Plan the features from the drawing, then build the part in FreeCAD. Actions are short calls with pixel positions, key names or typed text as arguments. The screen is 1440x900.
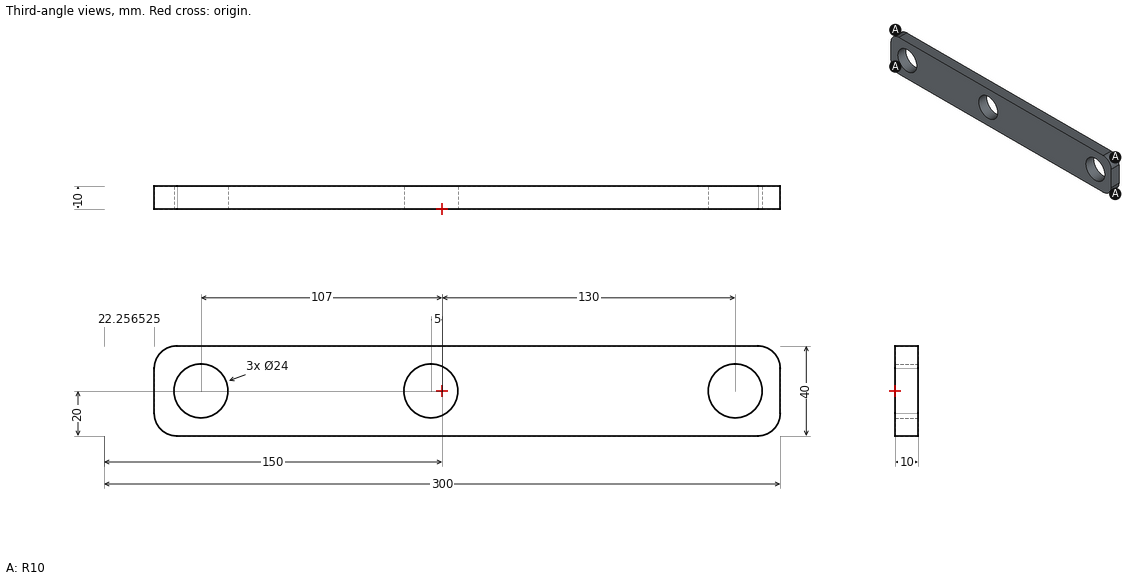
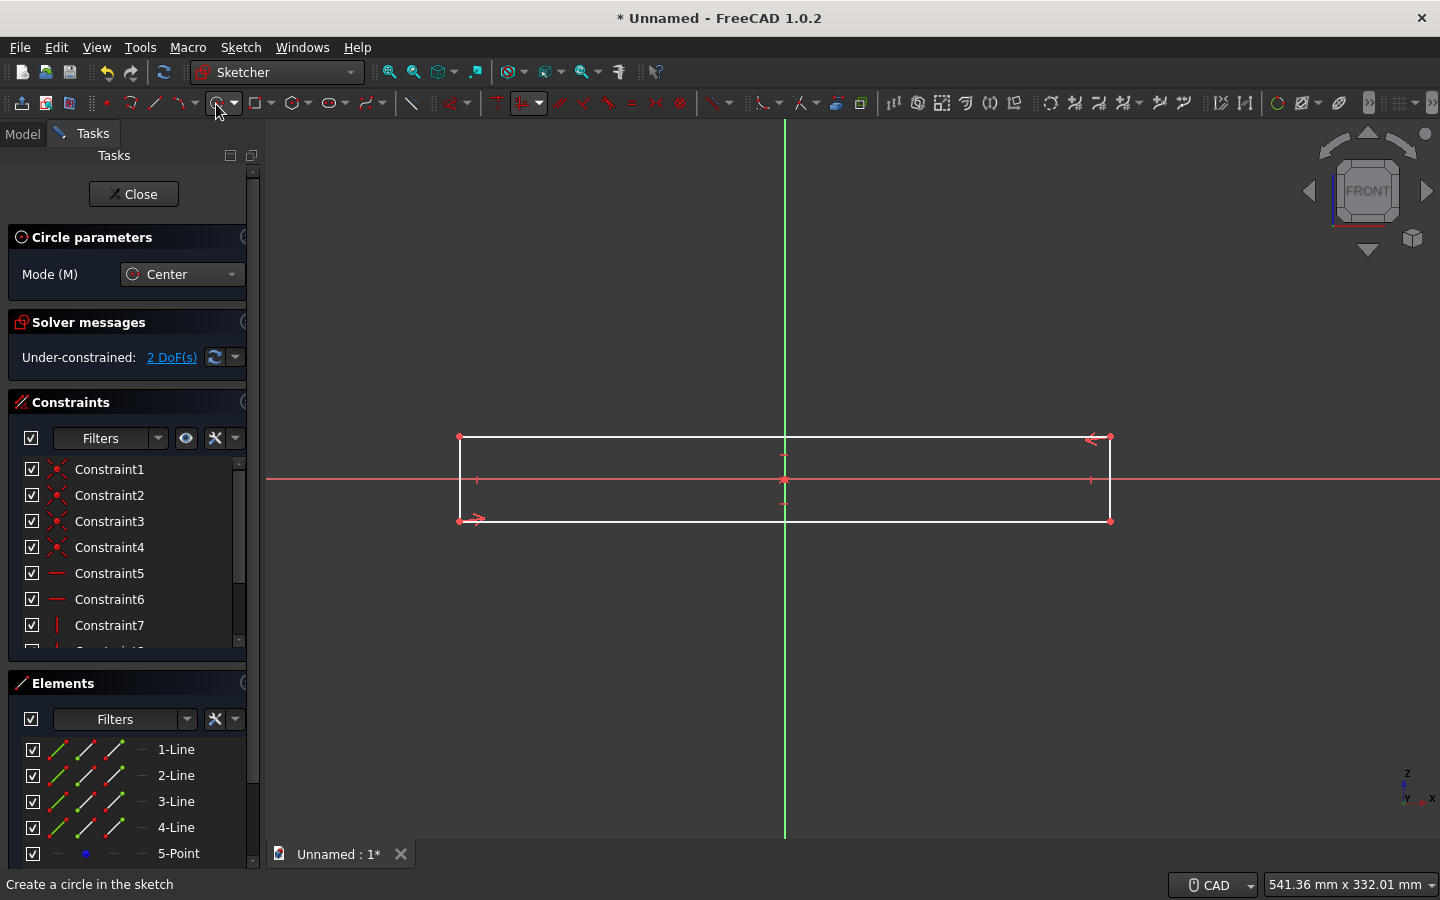
click(553, 479)
click(571, 461)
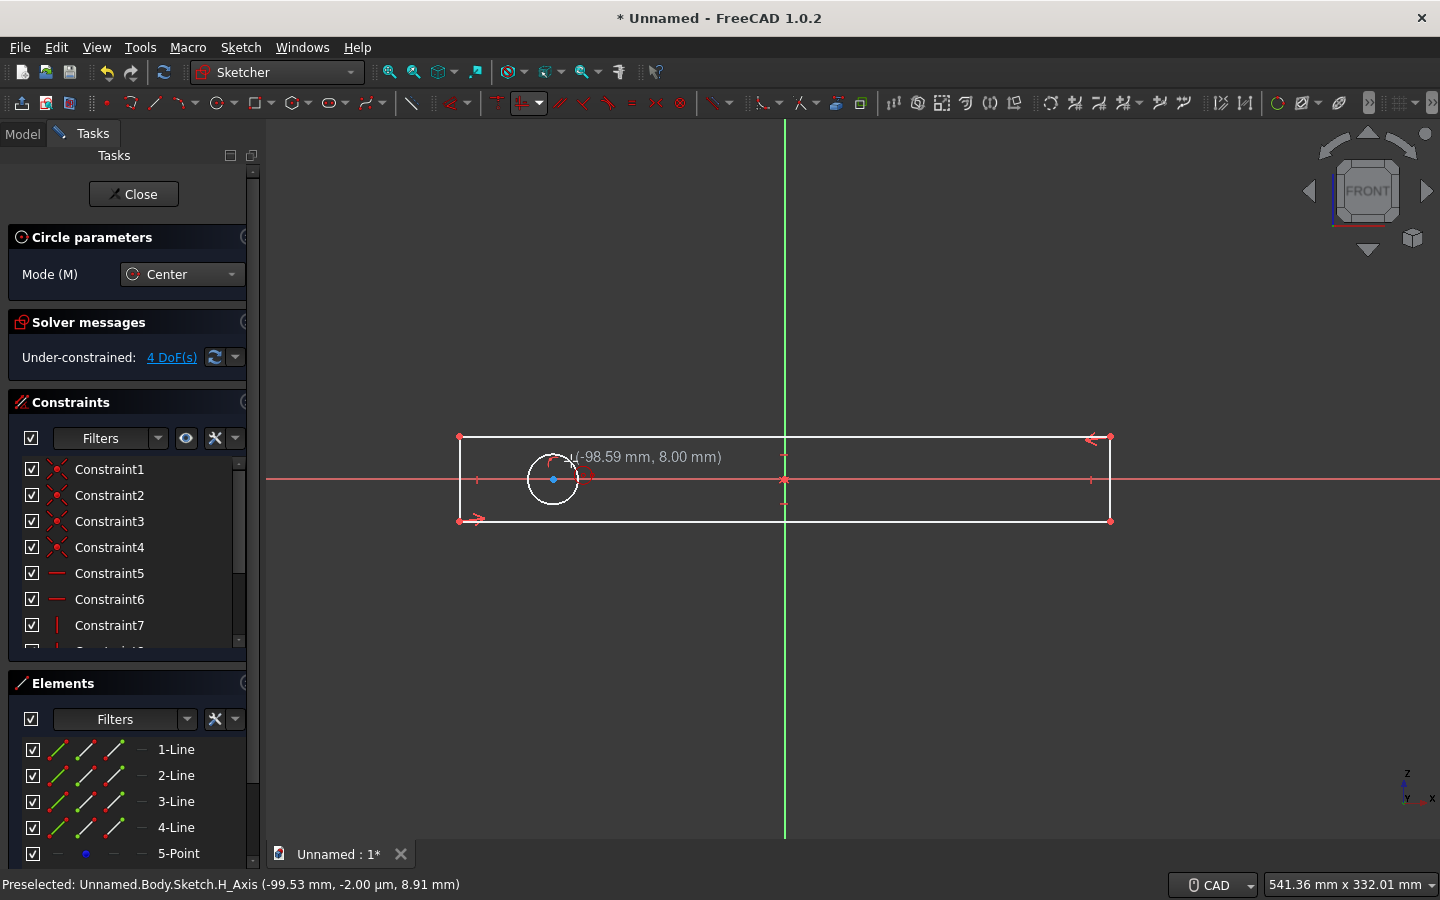
scroll(774, 479, up, 2)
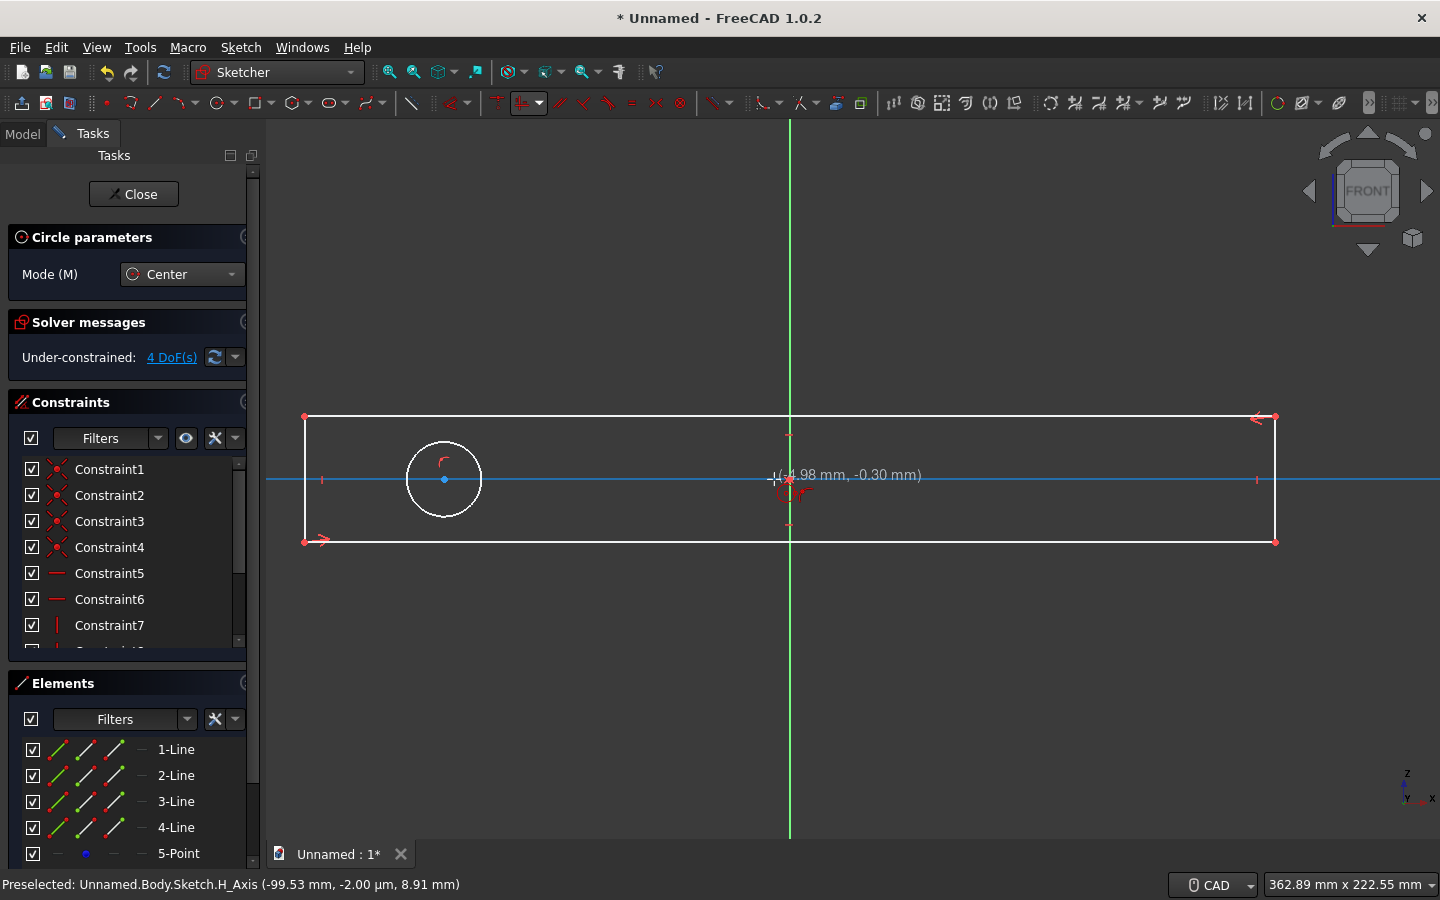
click(774, 479)
click(746, 452)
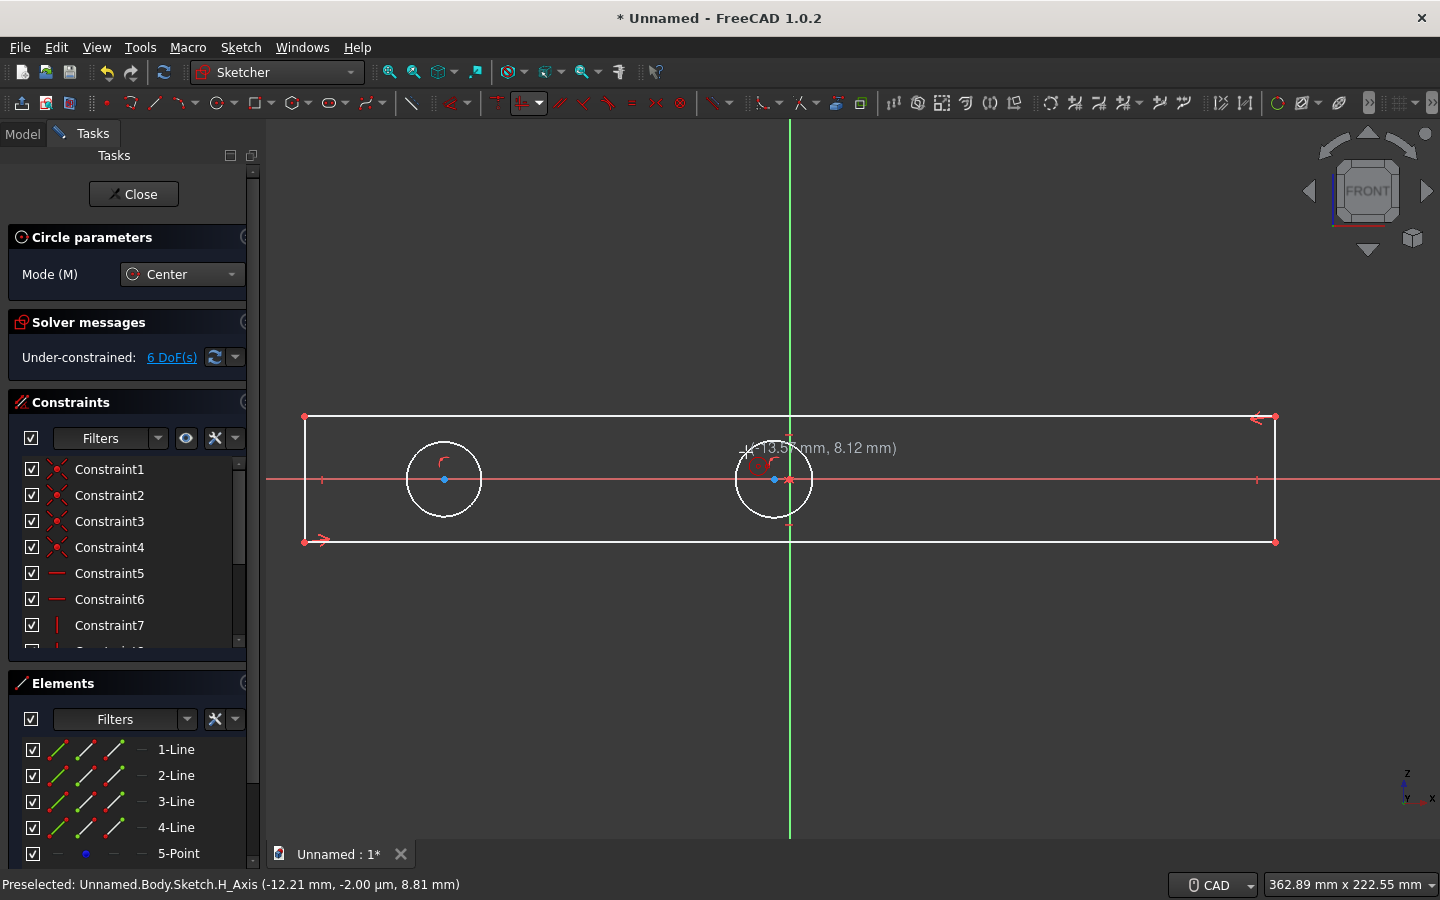
click(1210, 479)
click(1238, 452)
key(Escape)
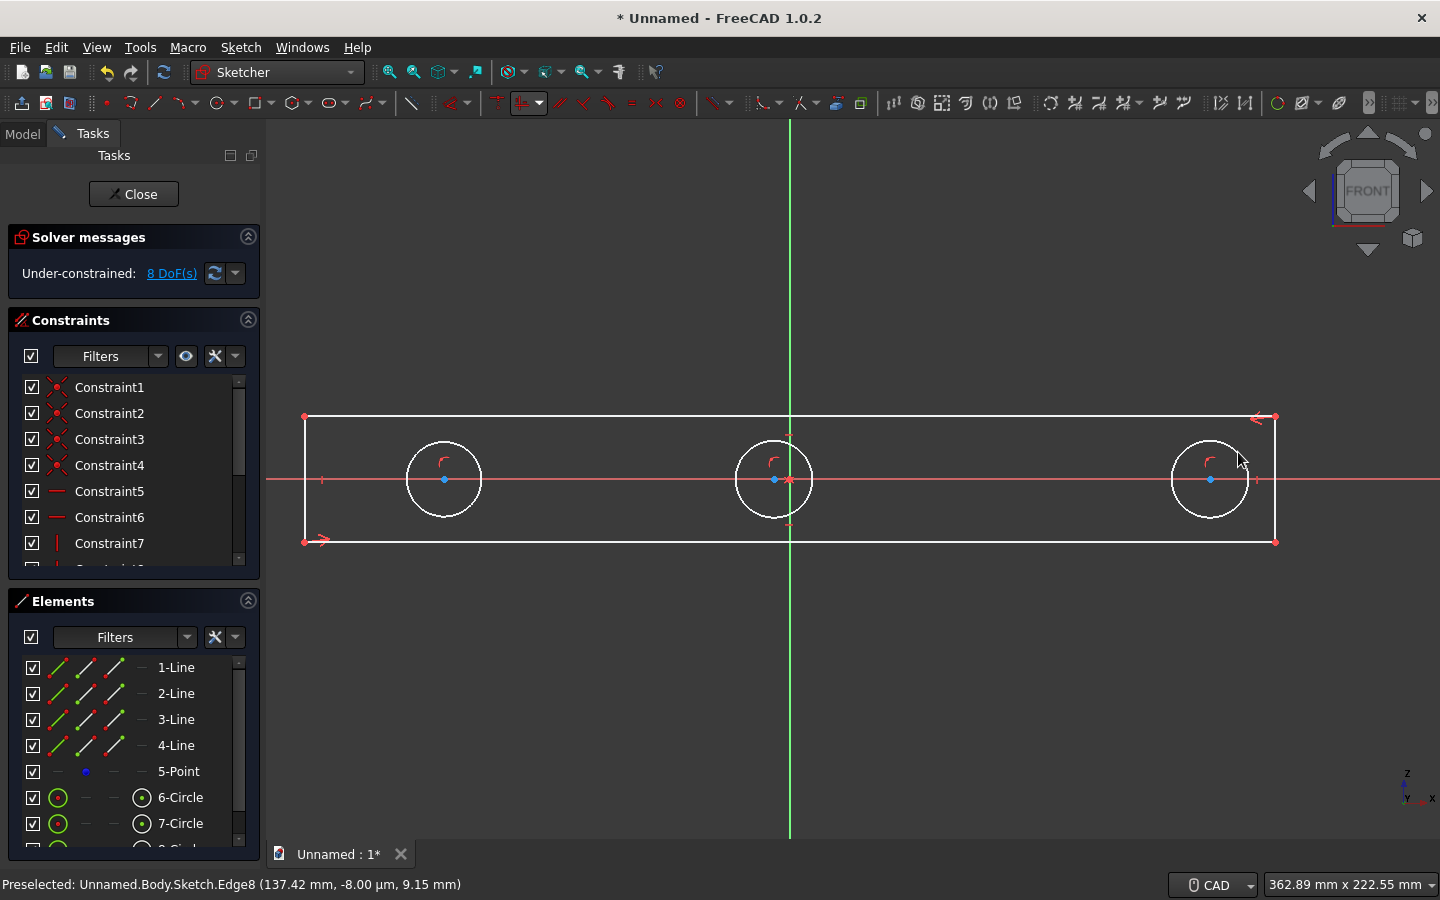
click(470, 453)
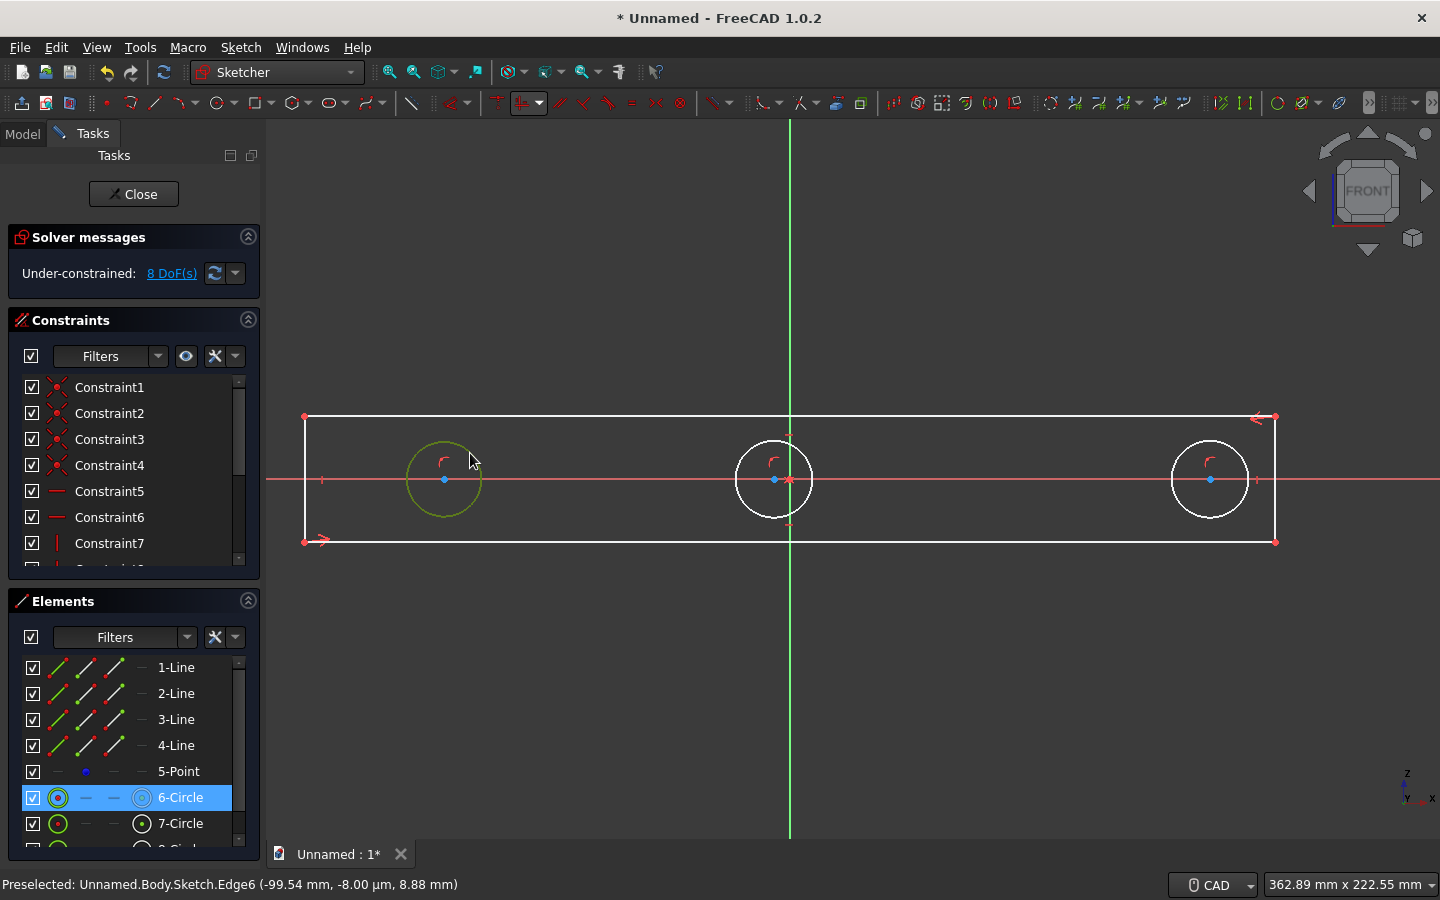
scroll(801, 452, up, 2)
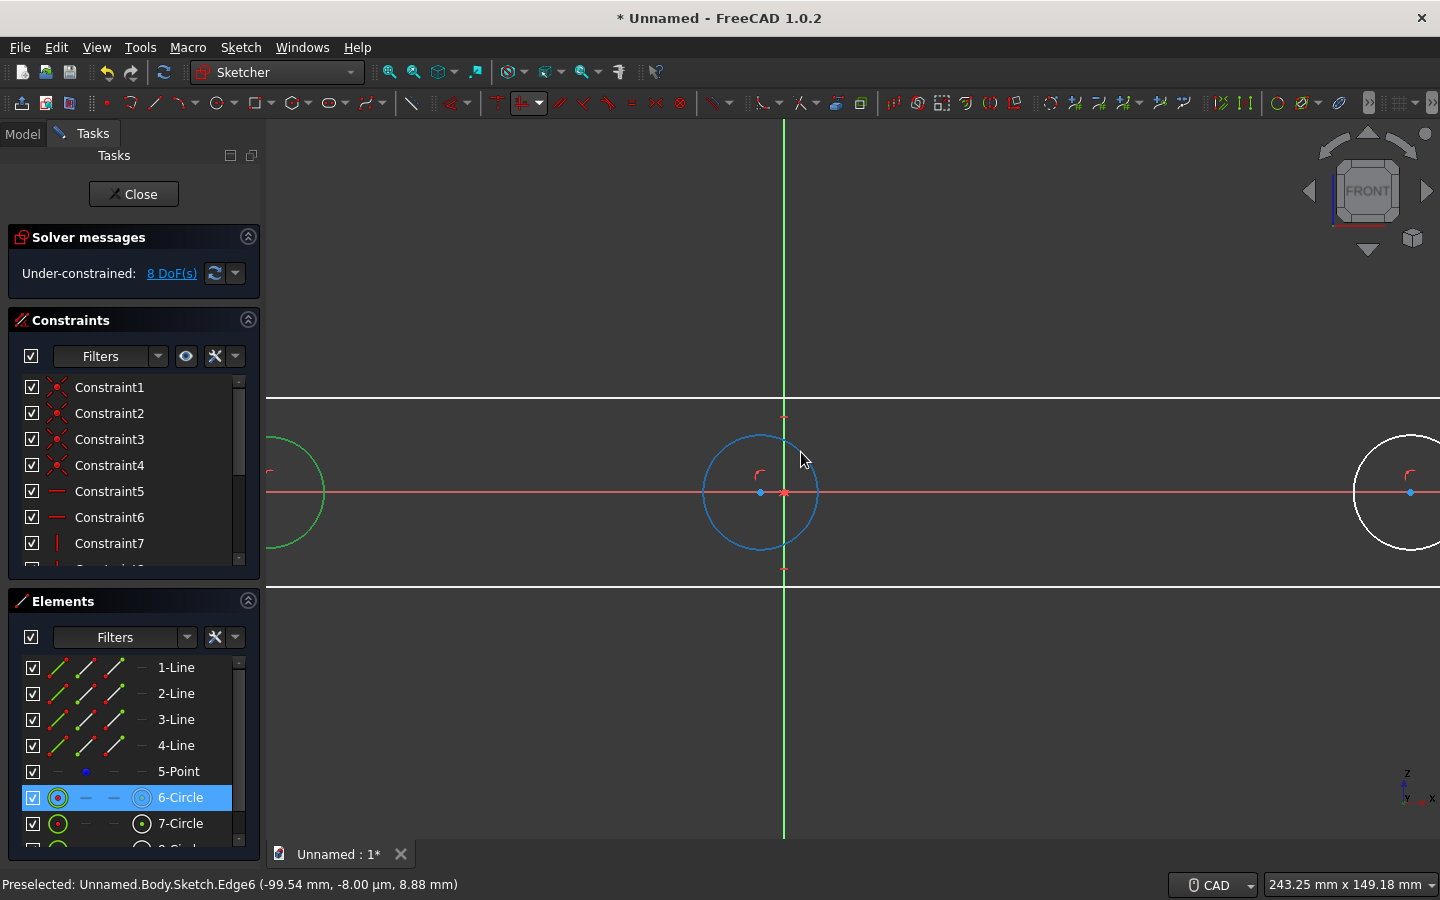
click(801, 452)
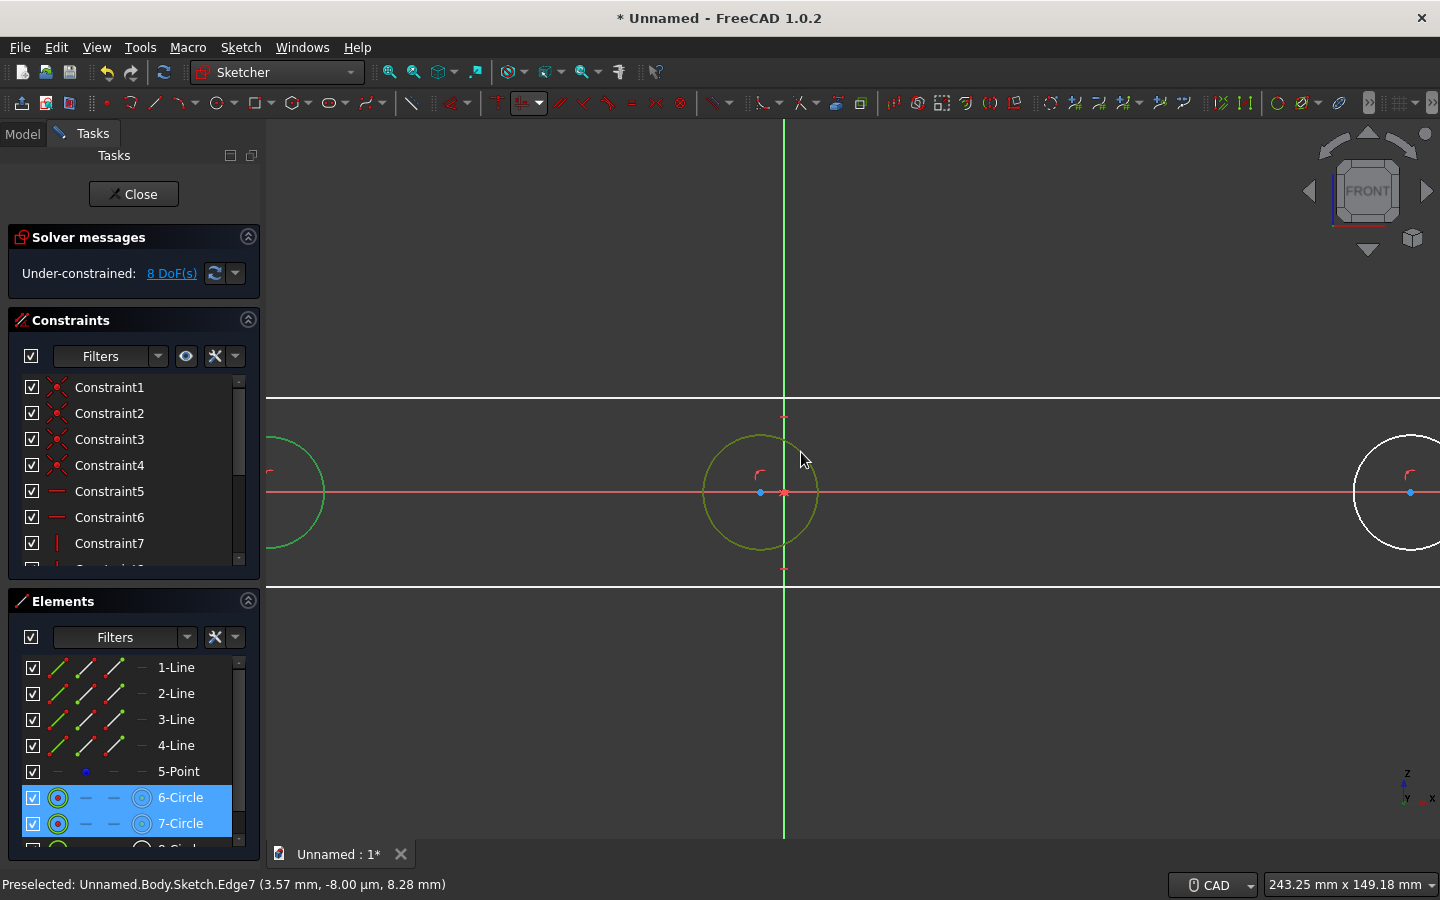
scroll(785, 468, down, 4)